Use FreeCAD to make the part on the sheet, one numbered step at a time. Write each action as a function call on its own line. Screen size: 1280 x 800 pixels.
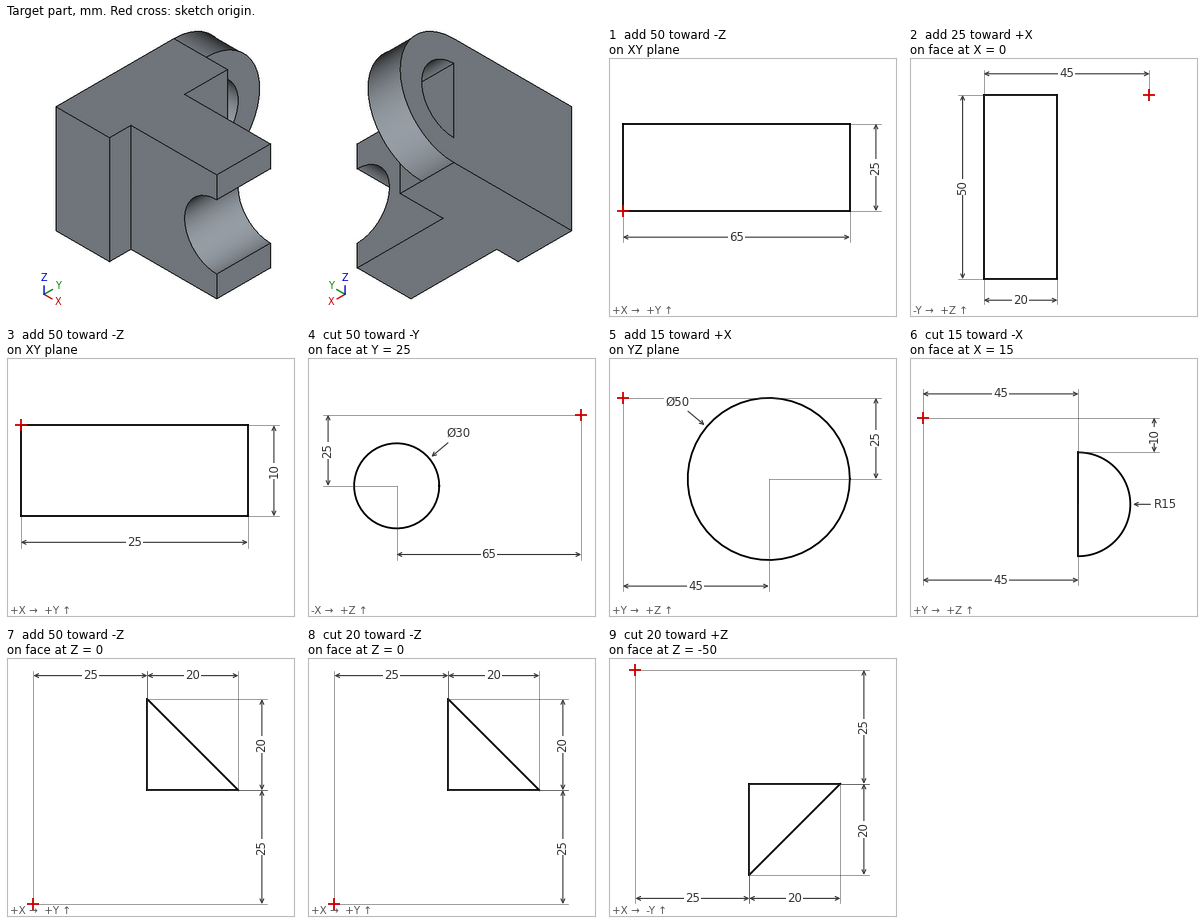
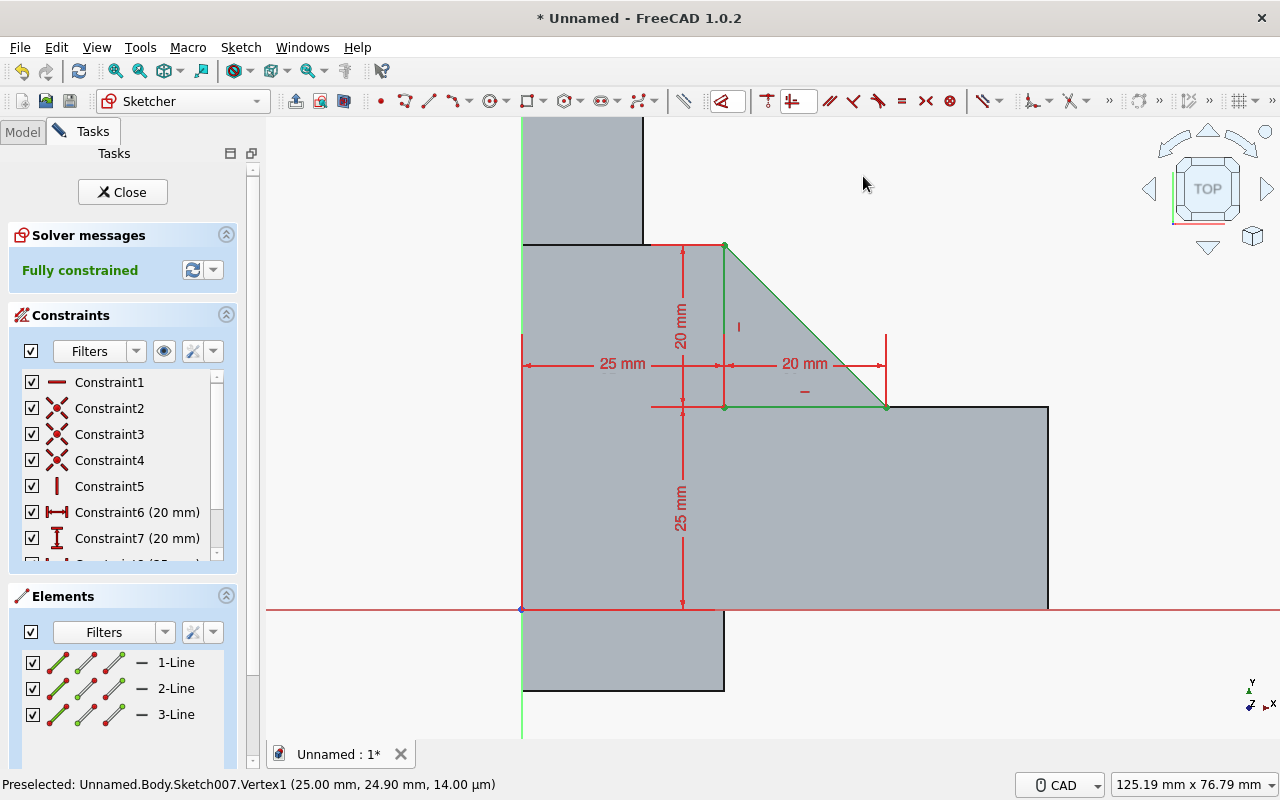
click(123, 192)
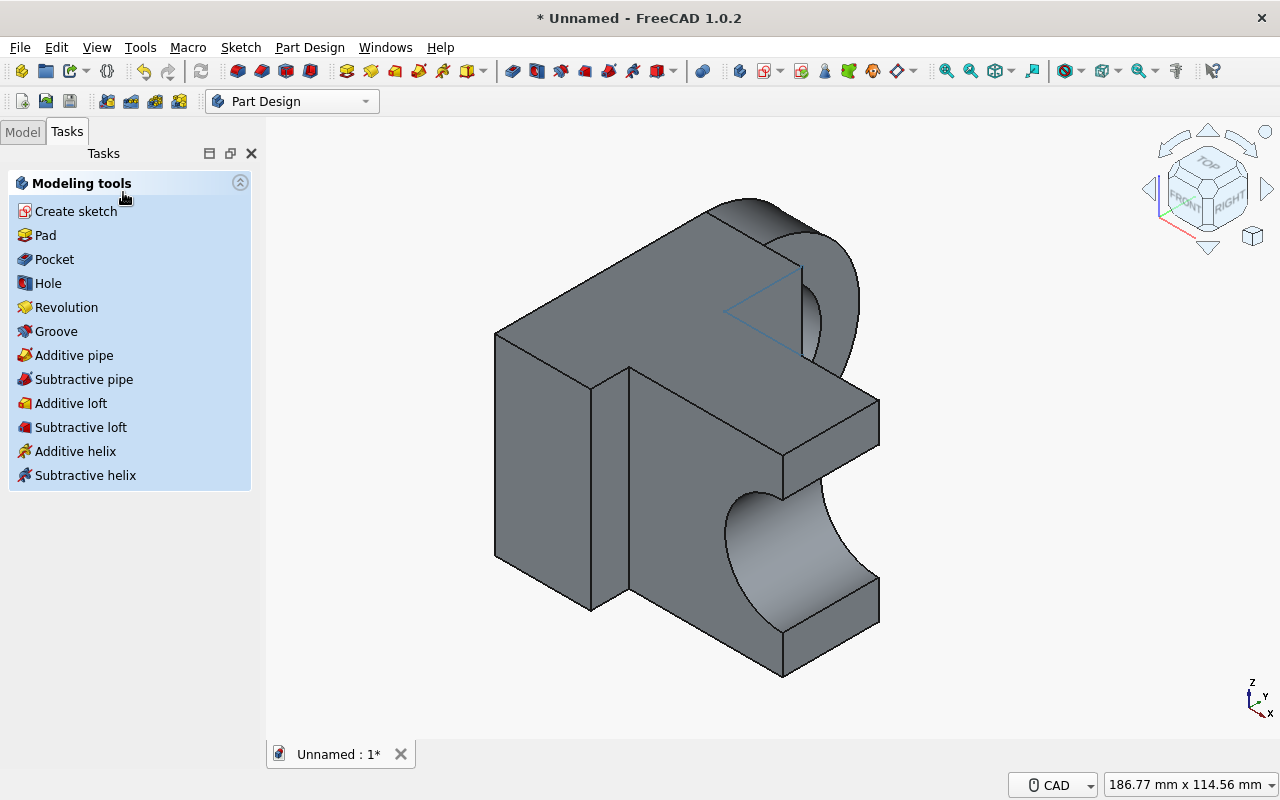
click(514, 72)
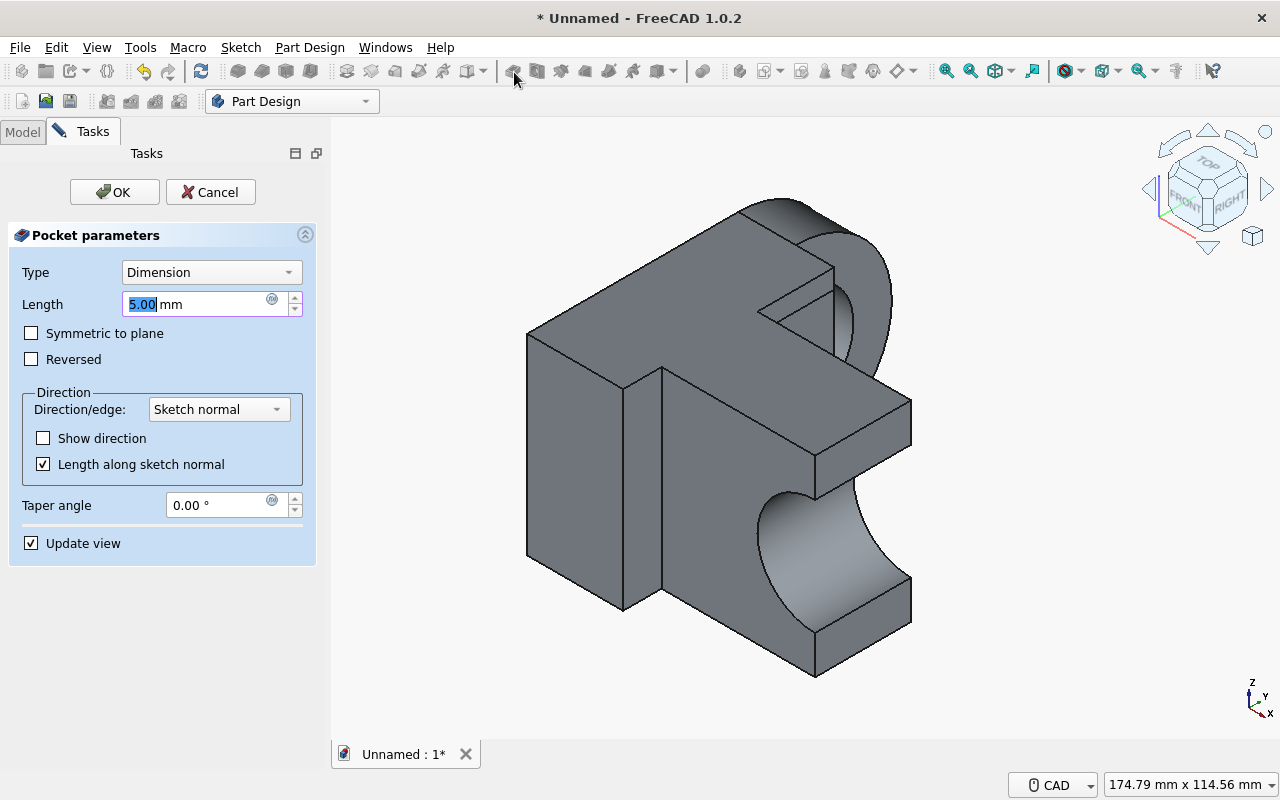
text(20)
key(Tab)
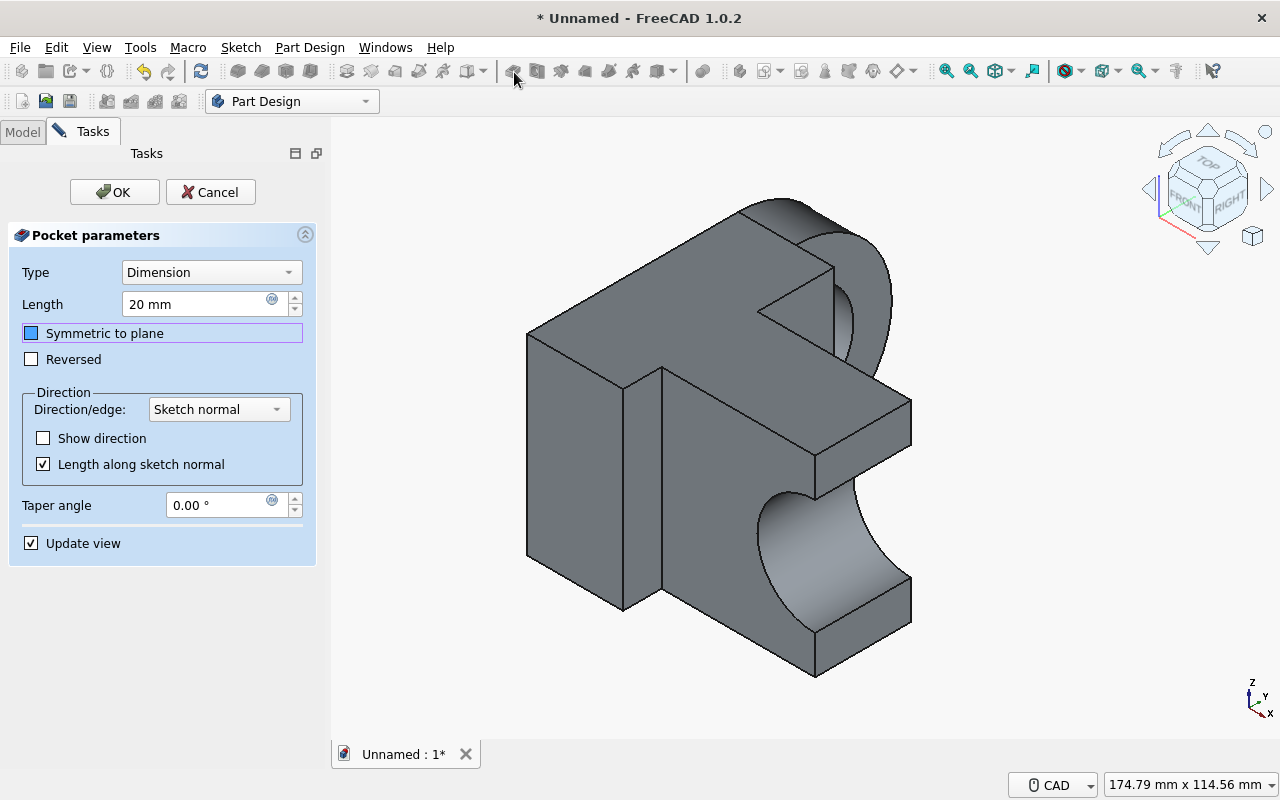
click(115, 192)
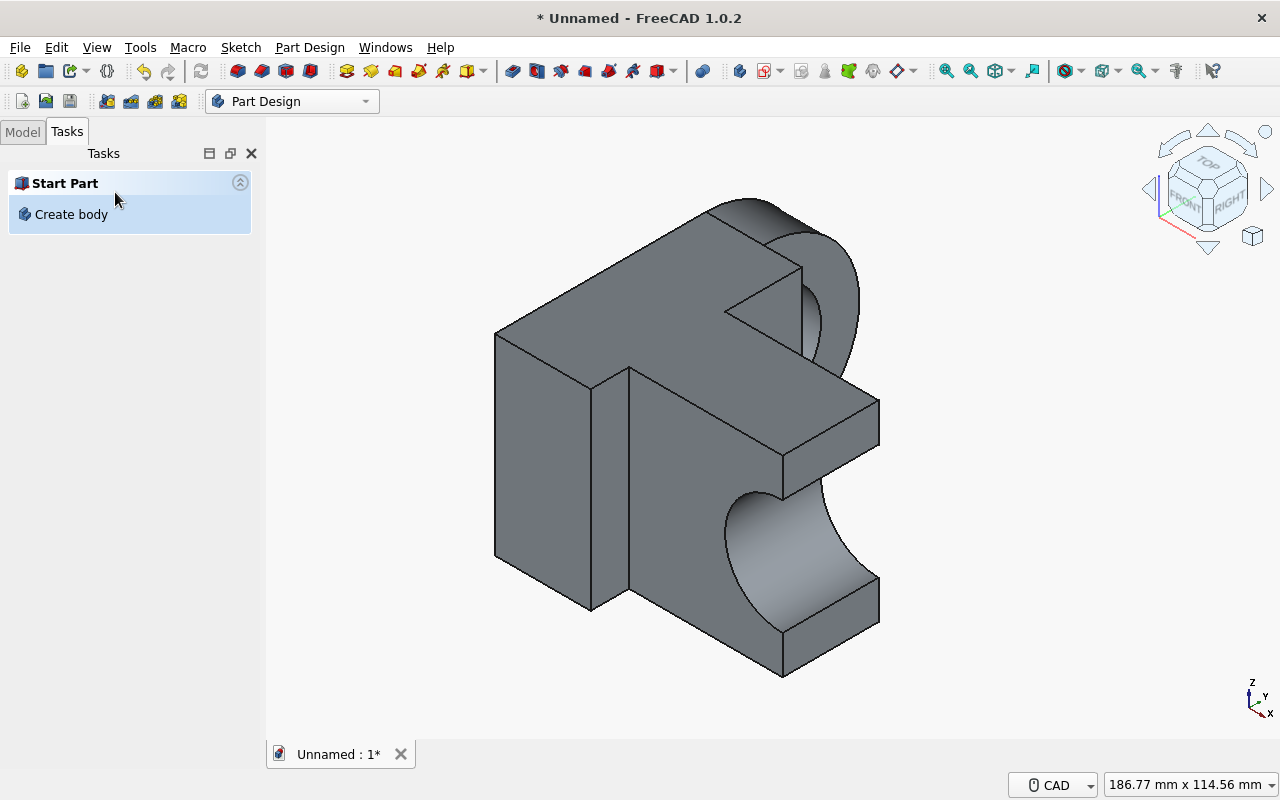
key(5)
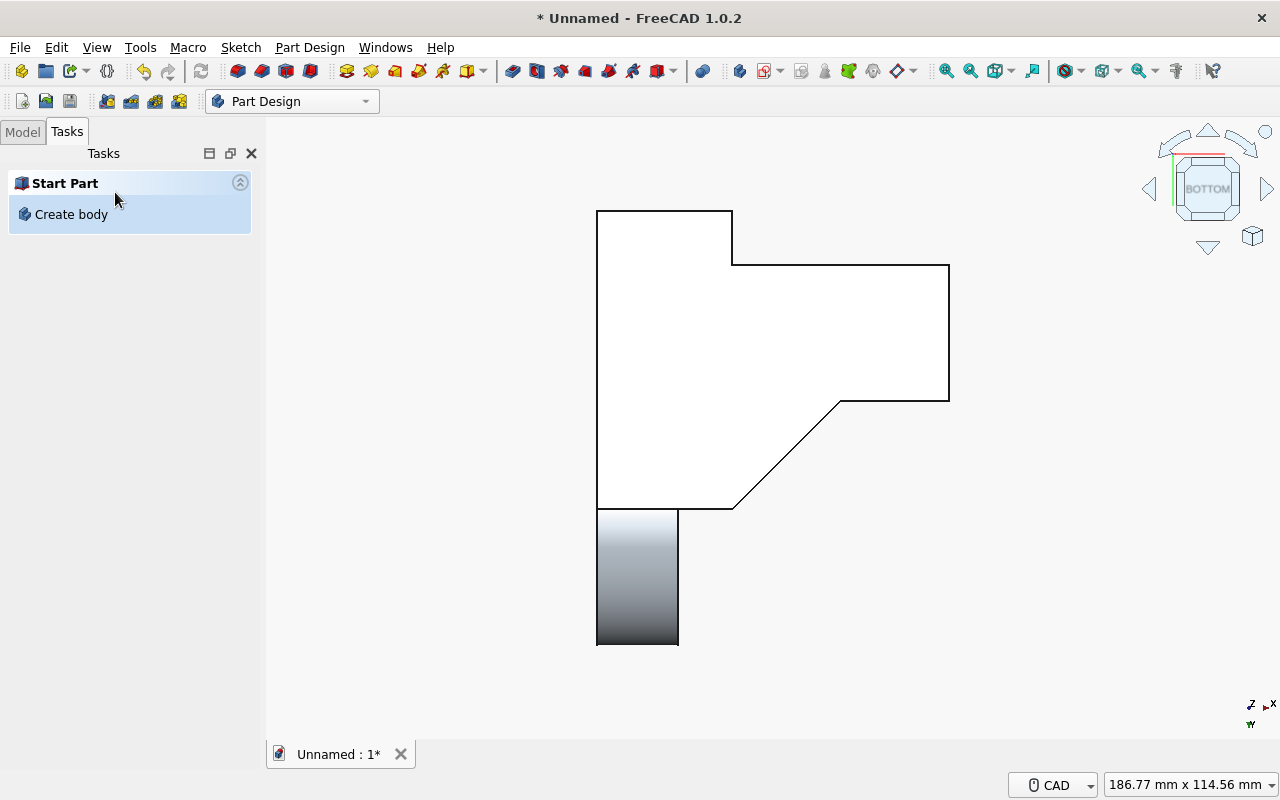
click(723, 359)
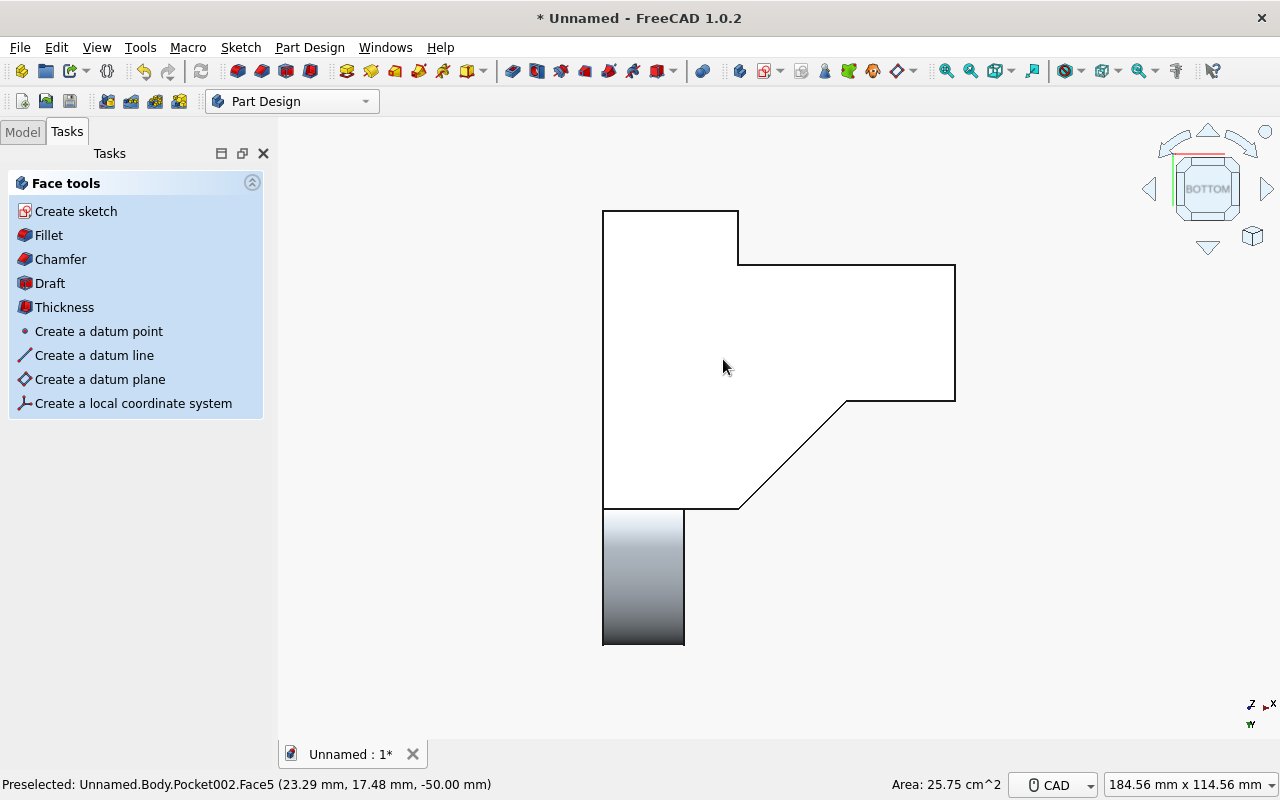
click(764, 72)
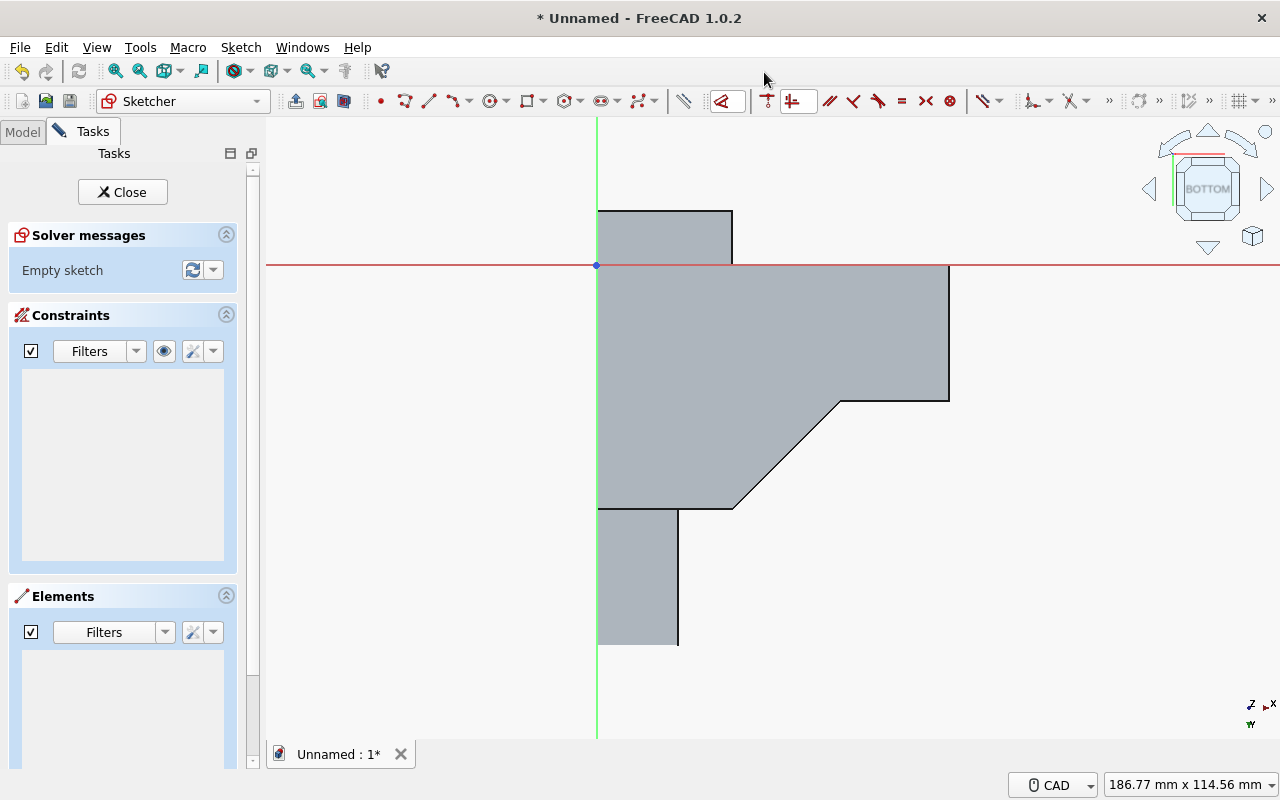
scroll(748, 304, up, 2)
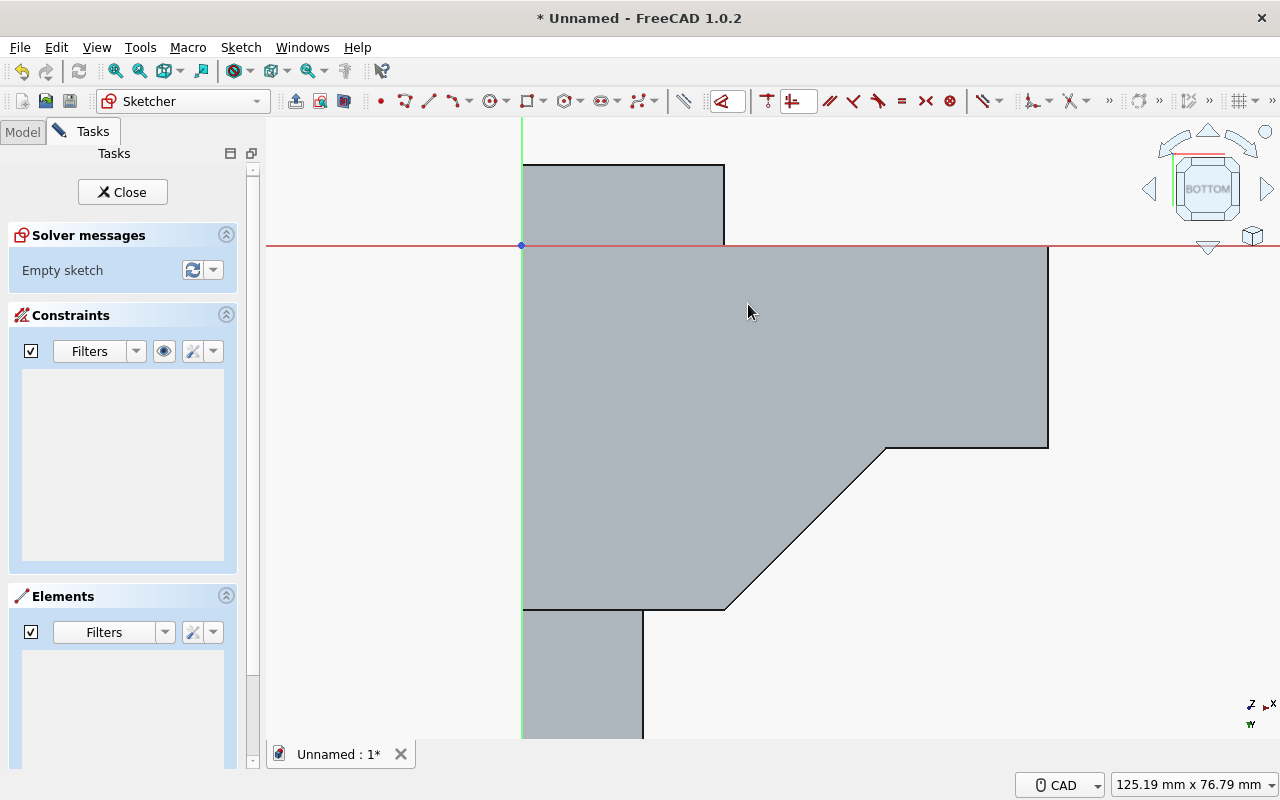
click(406, 102)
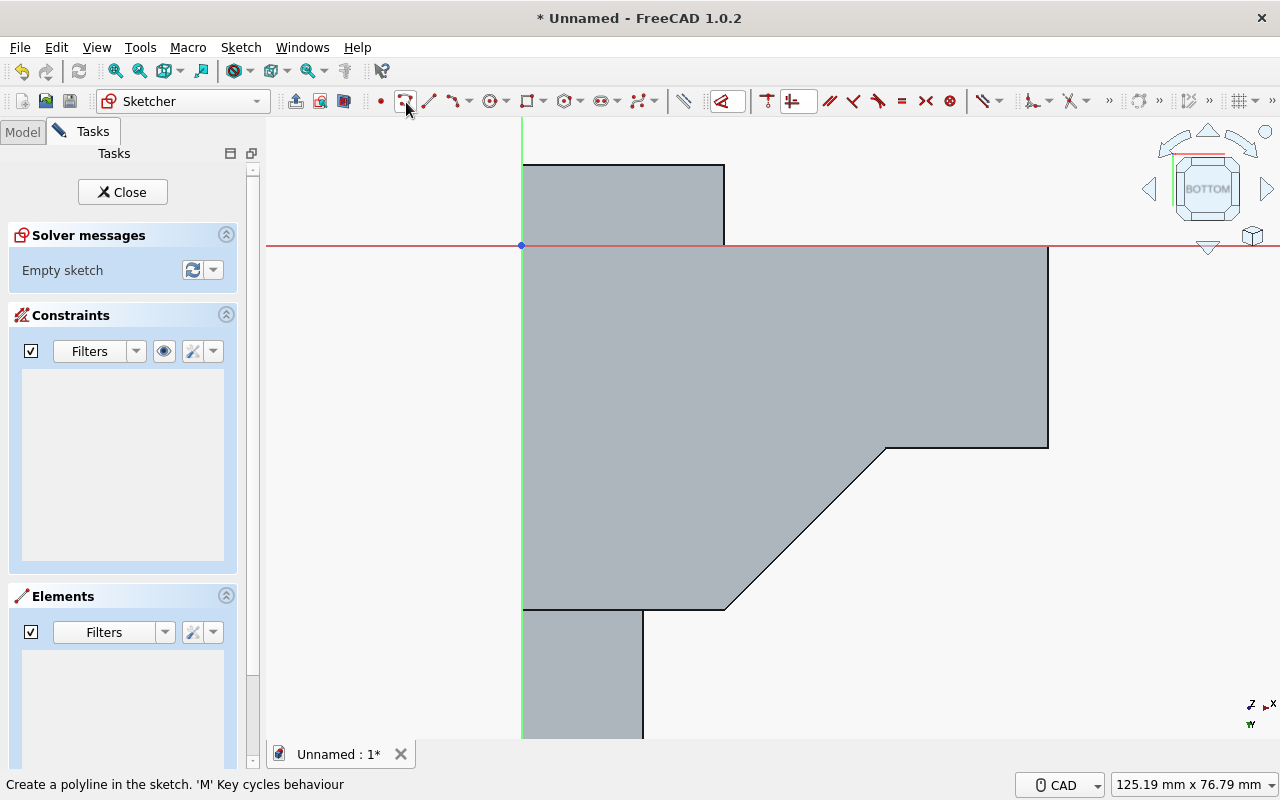
click(724, 448)
click(724, 610)
click(886, 448)
click(724, 449)
key(Escape)
key(Escape)